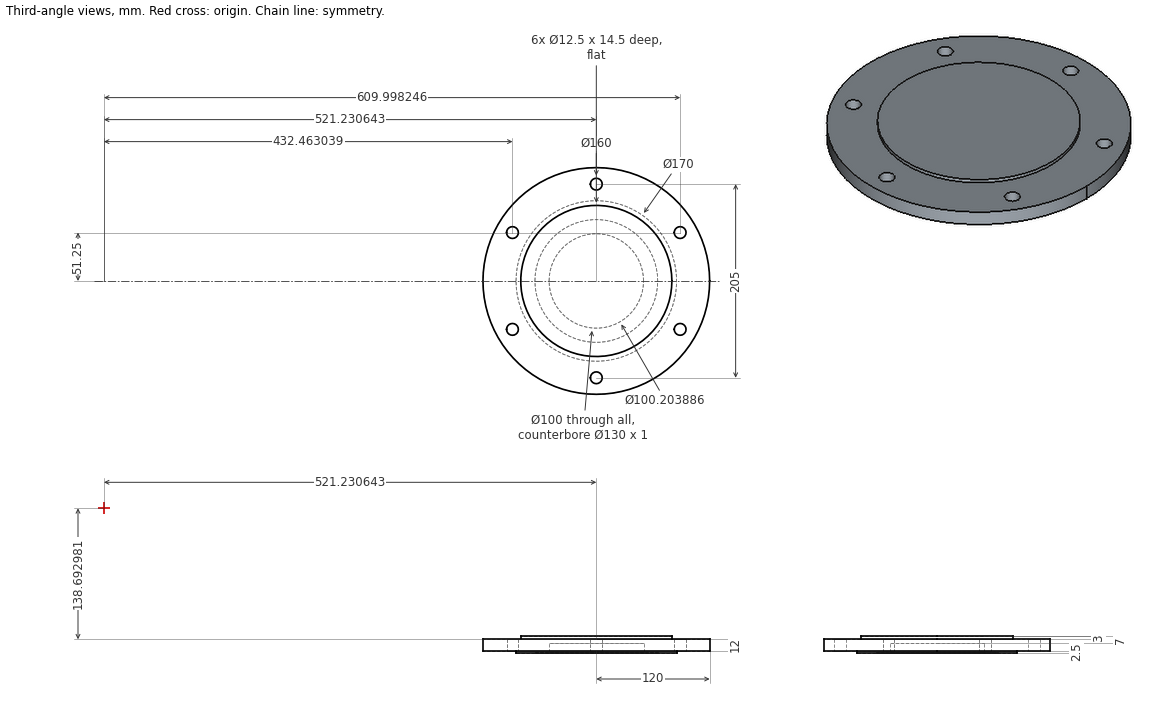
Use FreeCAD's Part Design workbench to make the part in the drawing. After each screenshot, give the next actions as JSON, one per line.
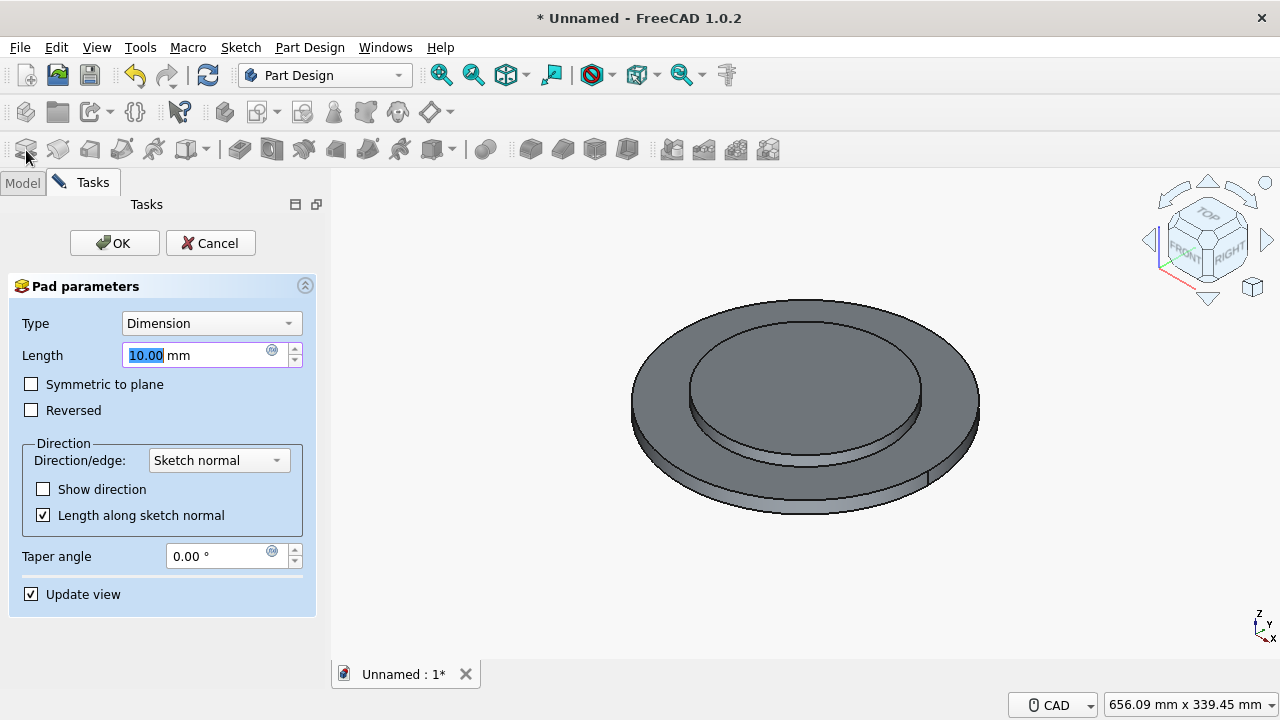
{"action": "type", "text": "3"}
{"action": "key", "text": "Tab"}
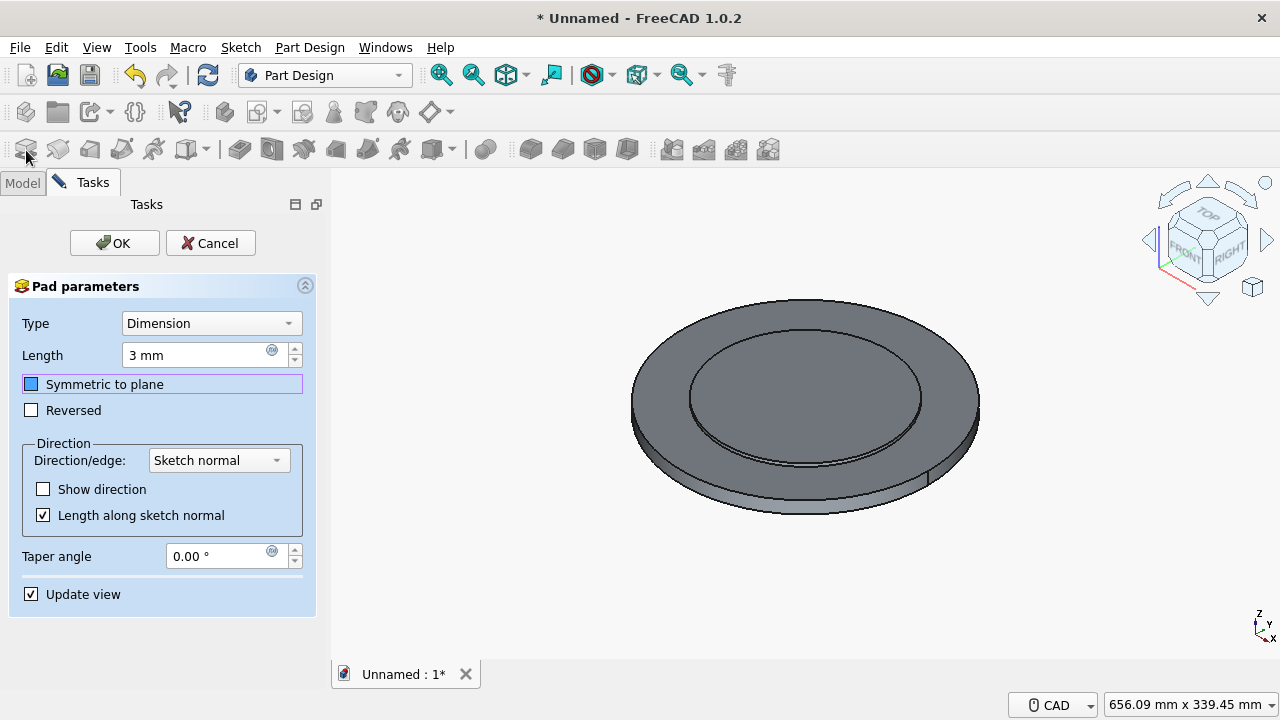
{"action": "left_click", "coordinate": [115, 243]}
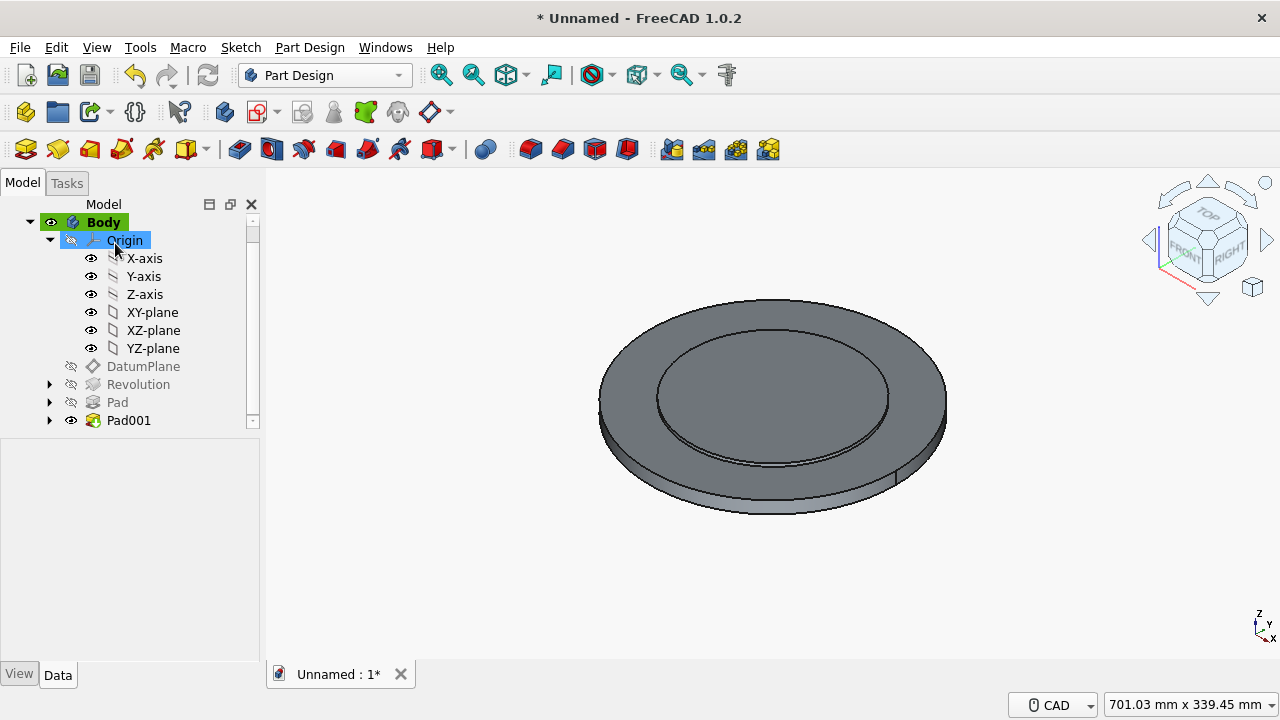
{"action": "left_click", "coordinate": [878, 338]}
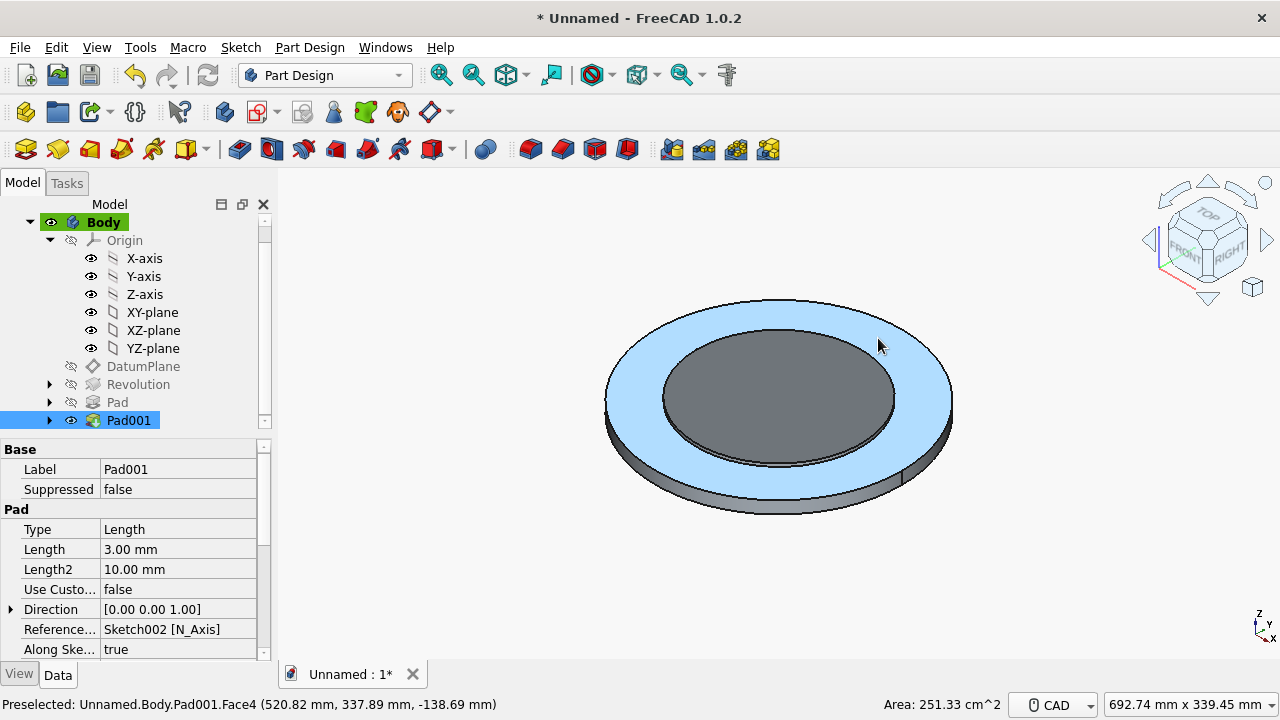
{"action": "left_click", "coordinate": [258, 112]}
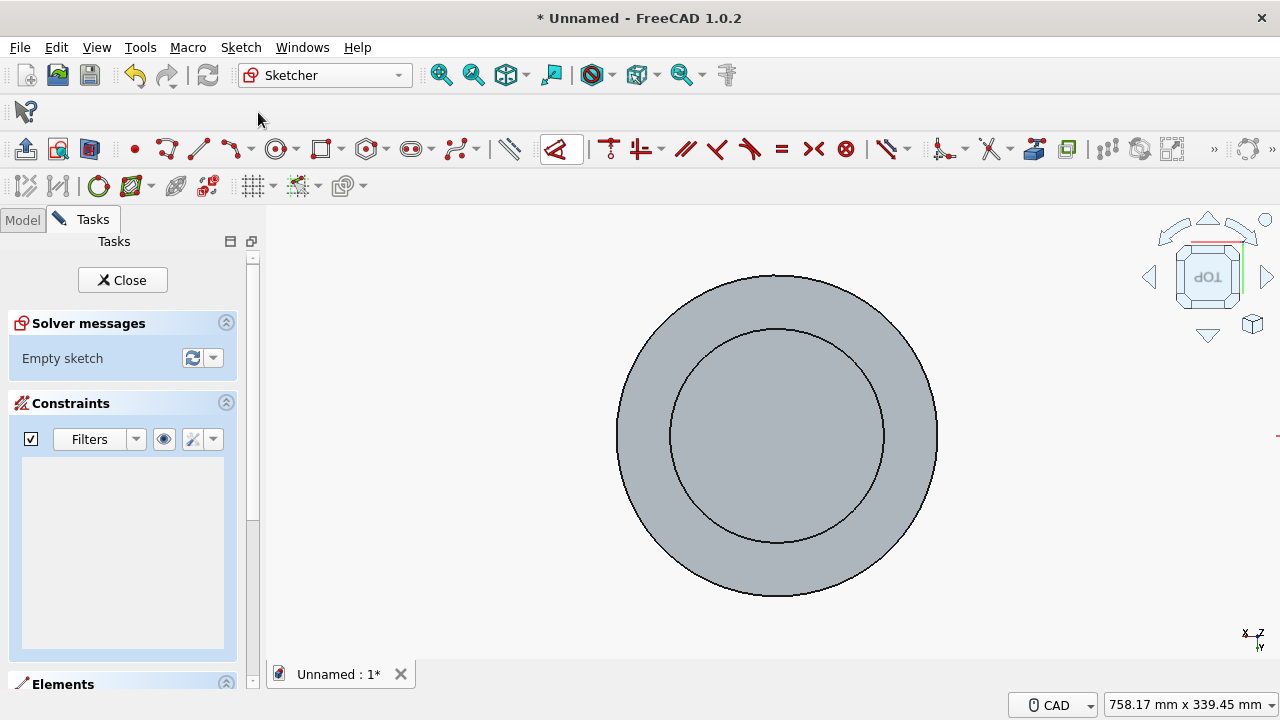
{"action": "key", "text": "g c"}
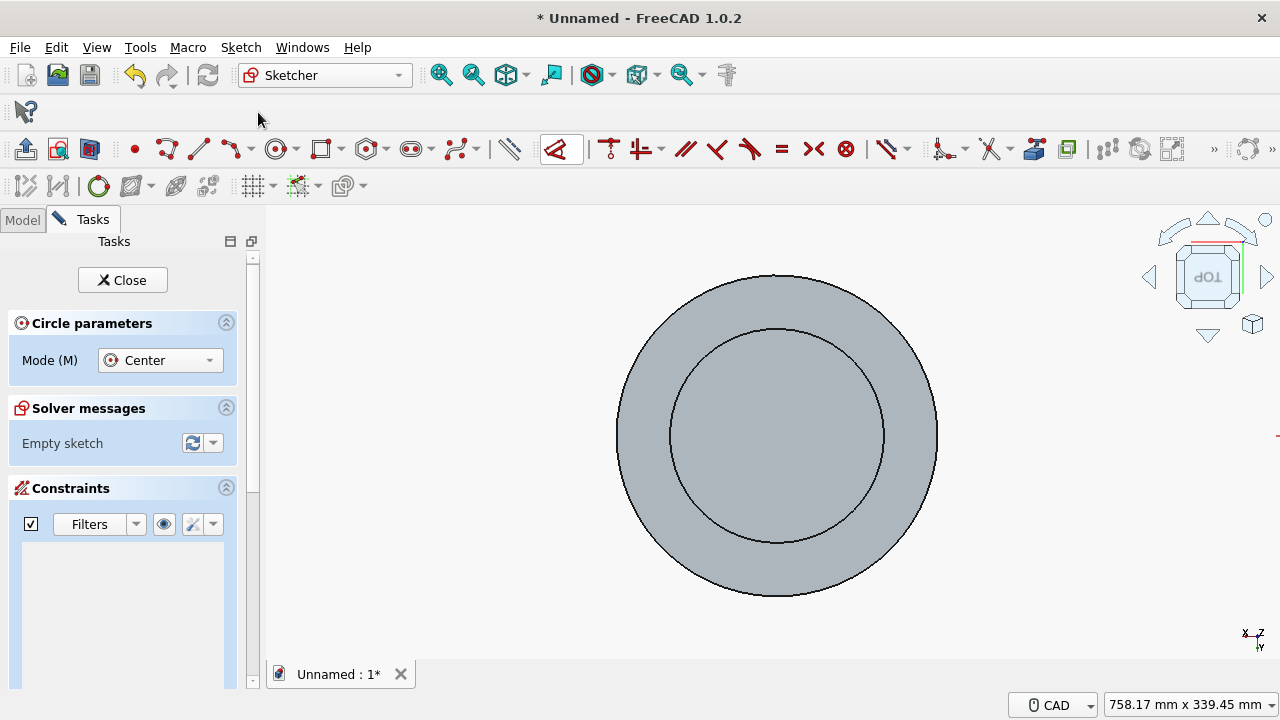
{"action": "scroll", "coordinate": [777, 573], "scroll_direction": "up", "scroll_amount": 5}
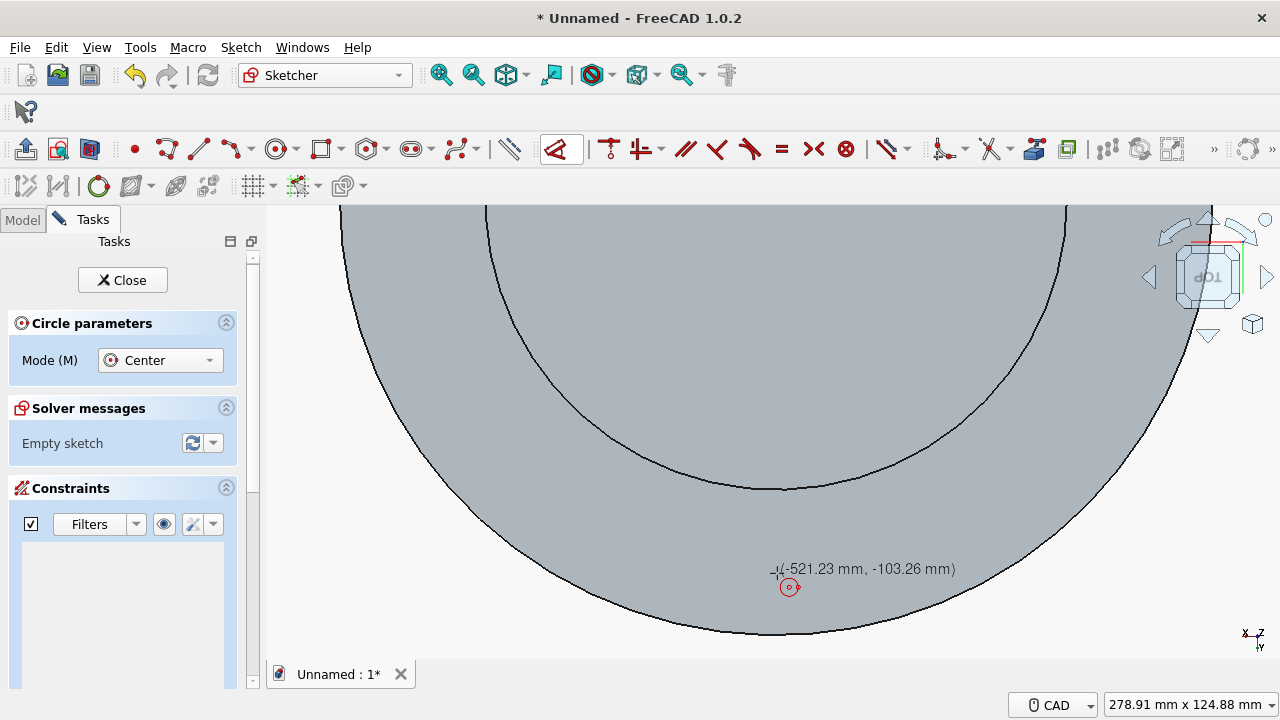
{"action": "left_click", "coordinate": [776, 572]}
{"action": "mouse_move", "coordinate": [792, 555]}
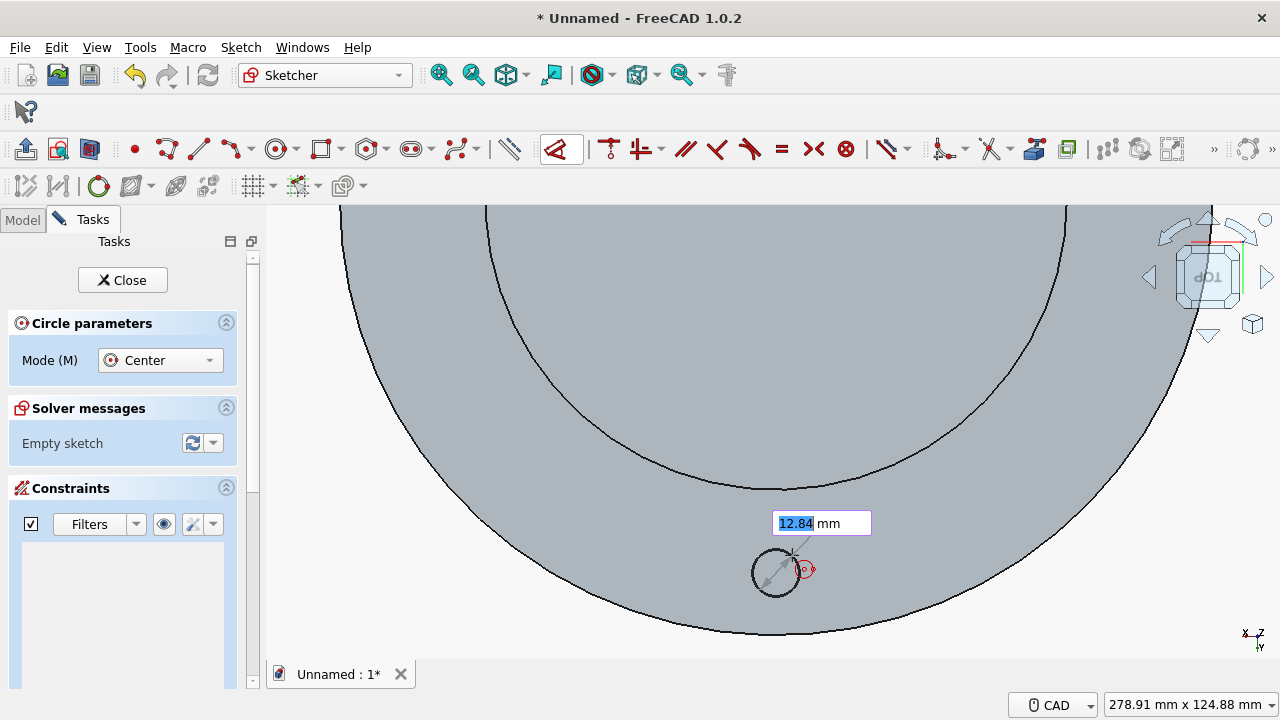
{"action": "type", "text": "12.5"}
{"action": "key", "text": "Return"}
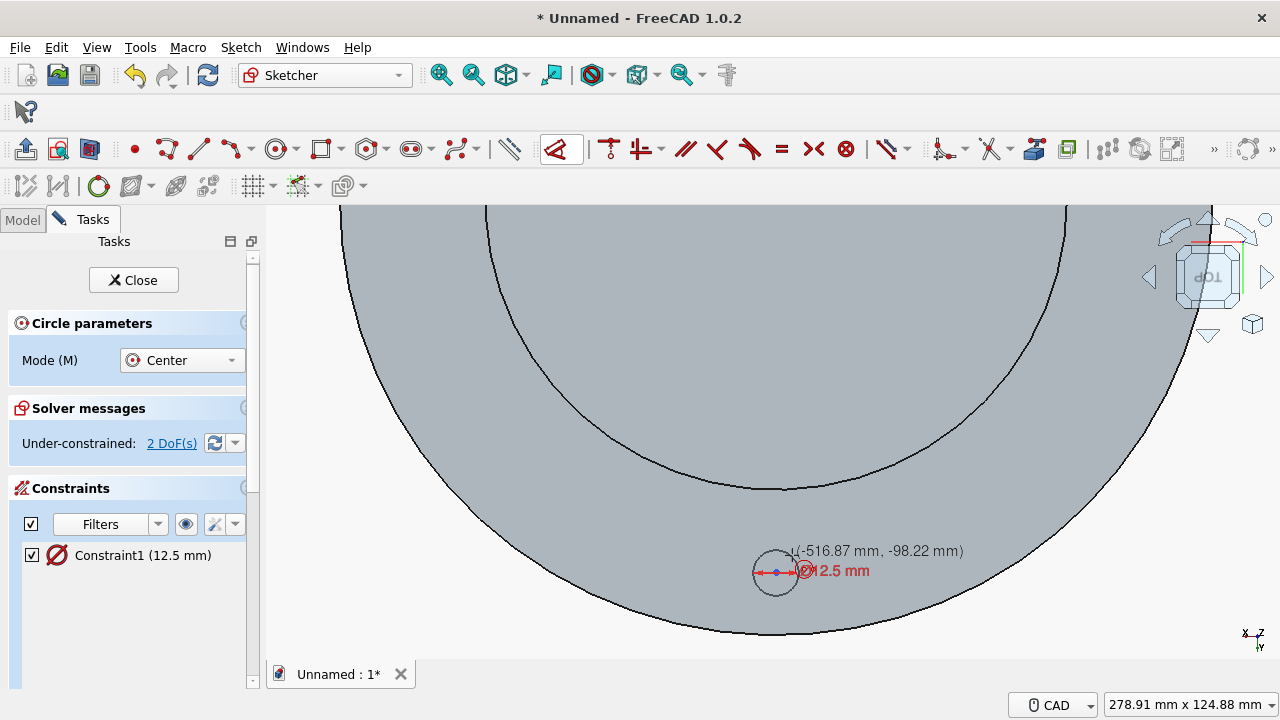
{"action": "left_click", "coordinate": [453, 385]}
{"action": "mouse_move", "coordinate": [469, 369]}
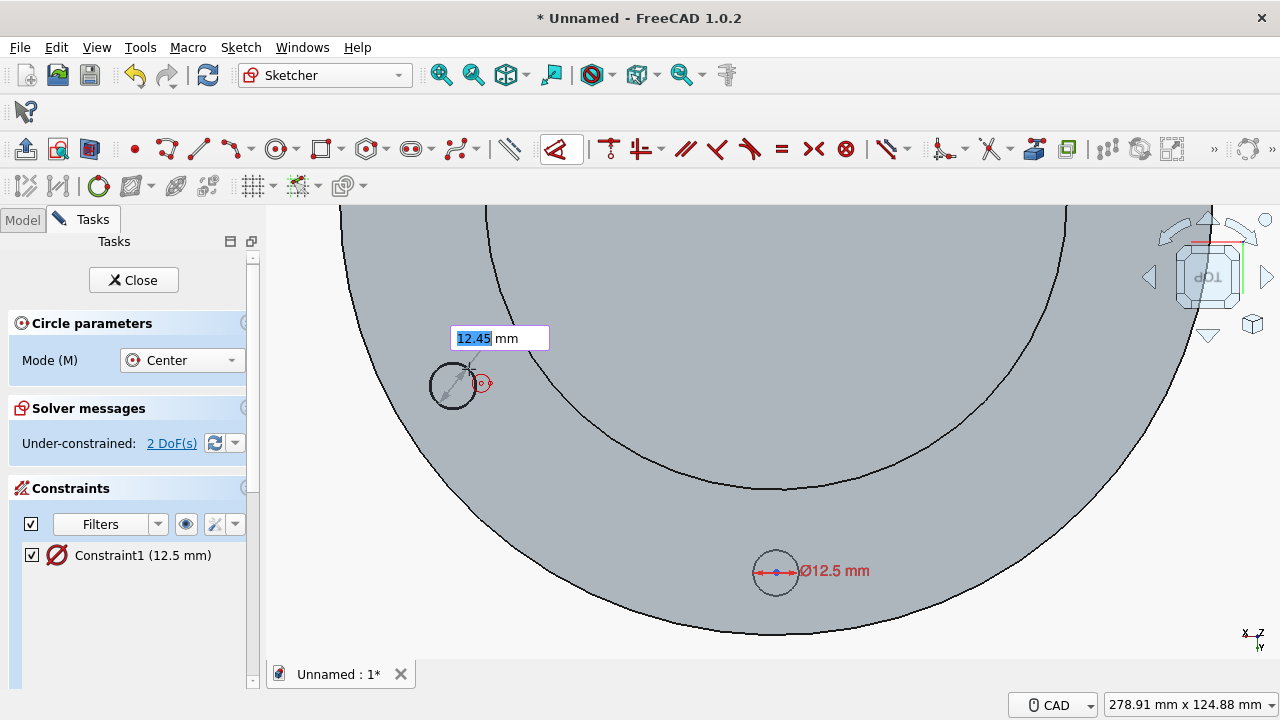
{"action": "type", "text": "12.5"}
{"action": "key", "text": "Return"}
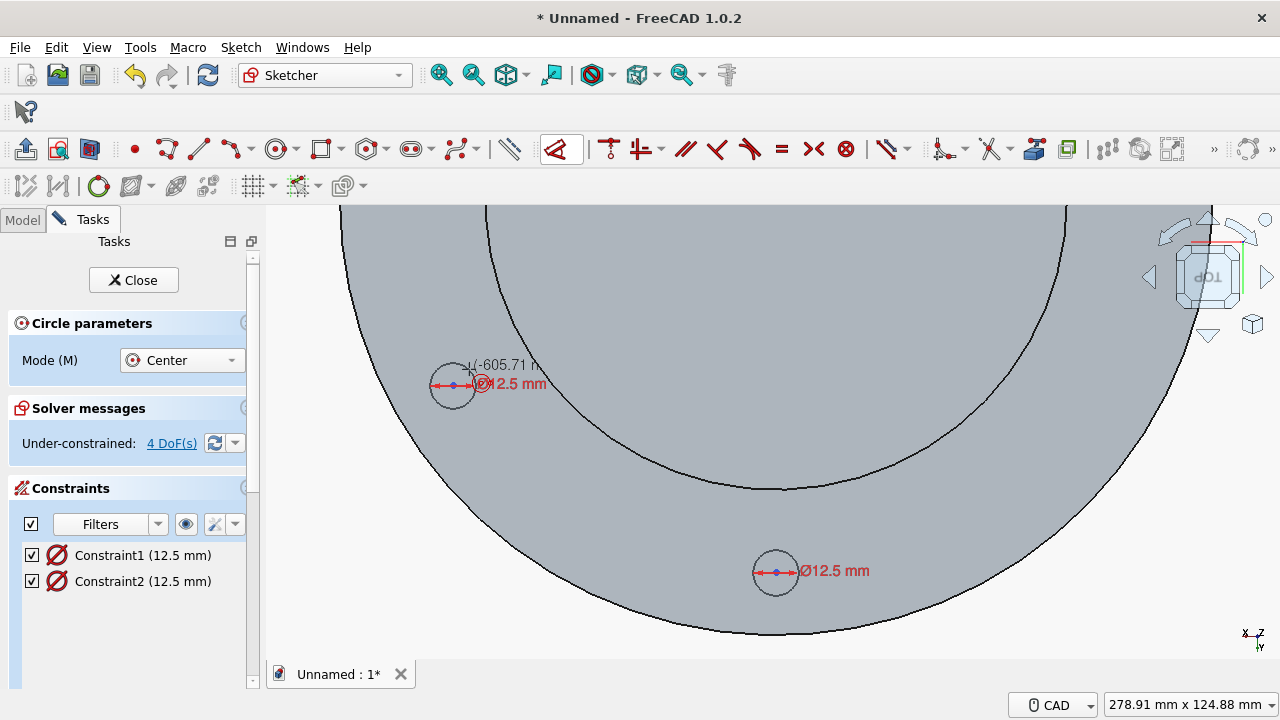
{"action": "left_click", "coordinate": [1099, 385]}
{"action": "mouse_move", "coordinate": [1115, 369]}